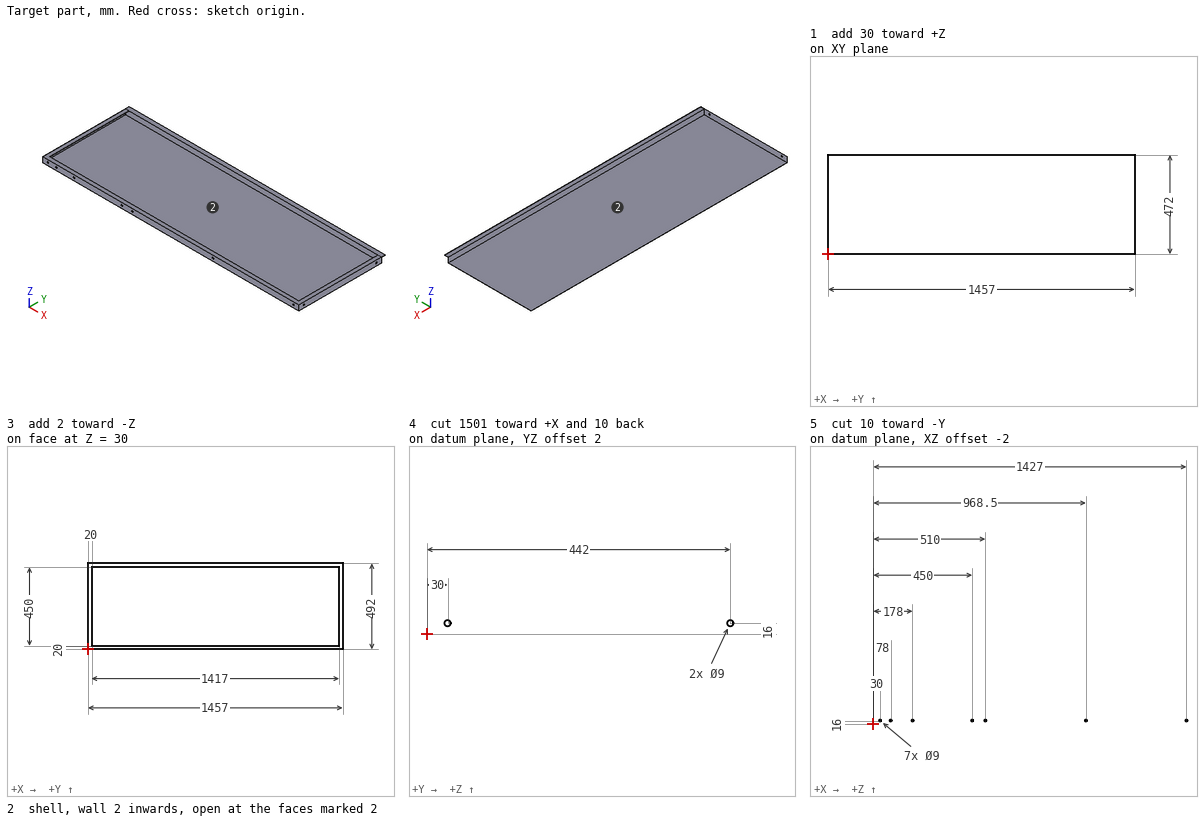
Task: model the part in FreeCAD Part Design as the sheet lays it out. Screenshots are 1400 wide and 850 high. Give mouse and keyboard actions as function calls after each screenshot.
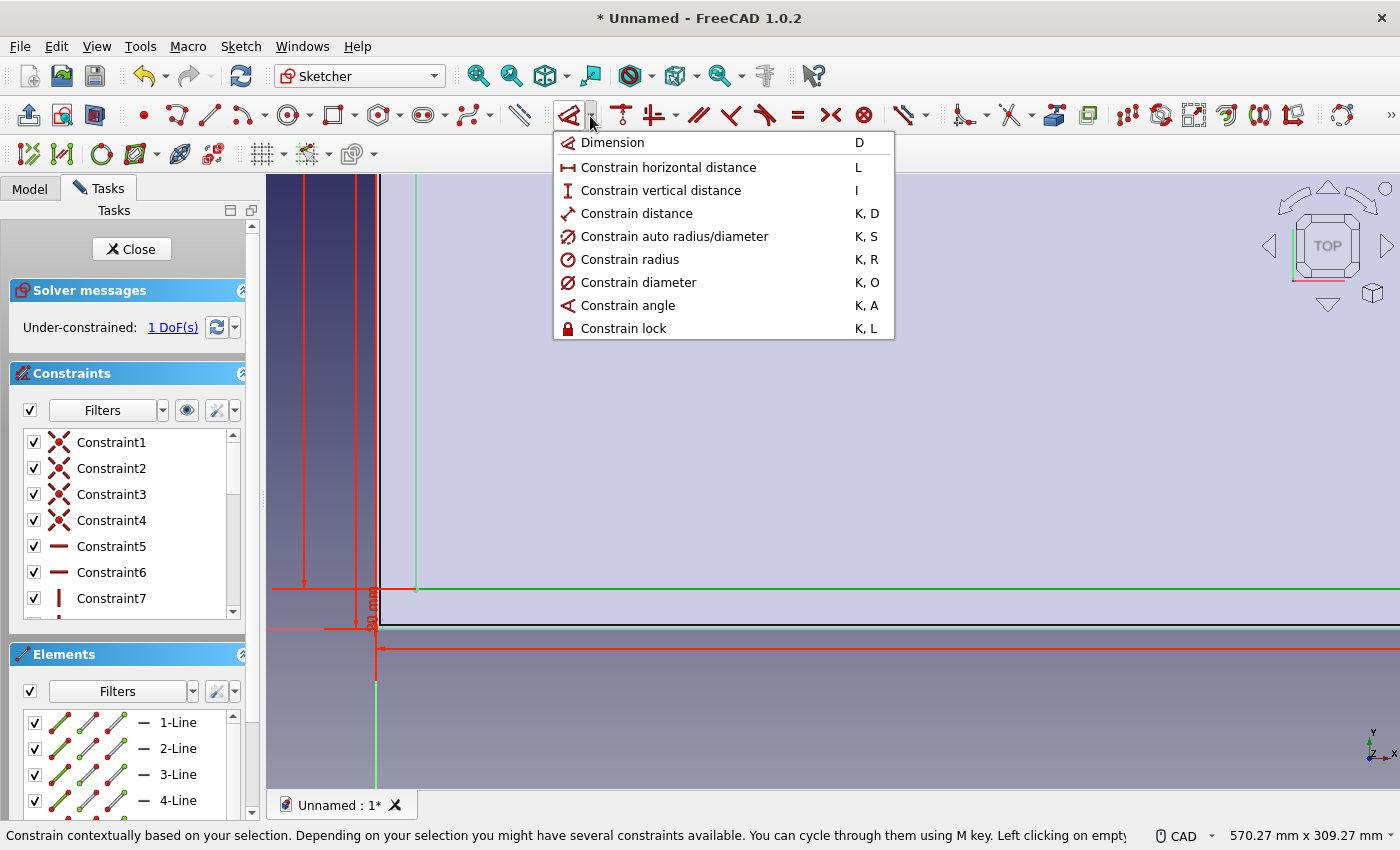
click(724, 168)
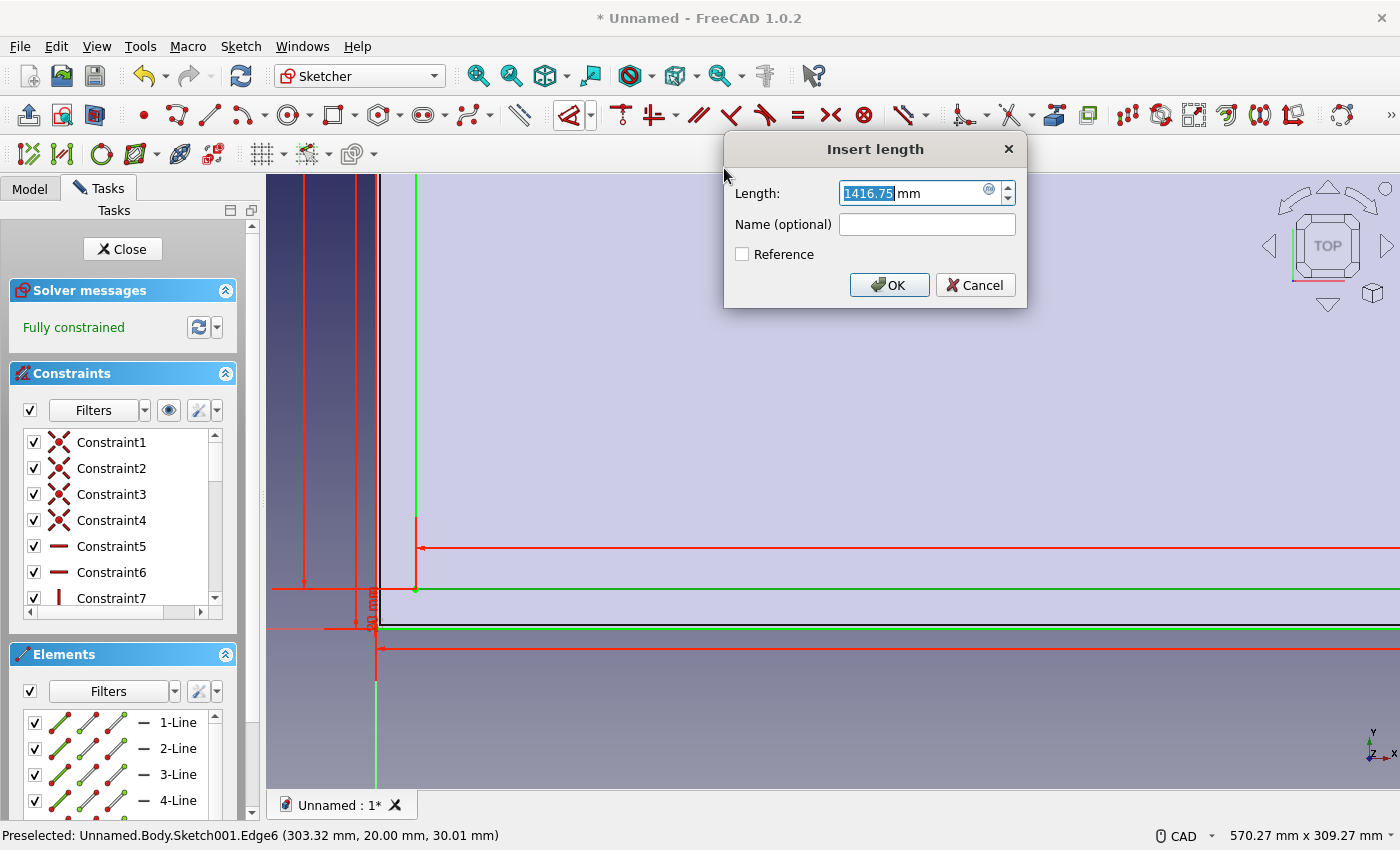
text(1417)
key(Return)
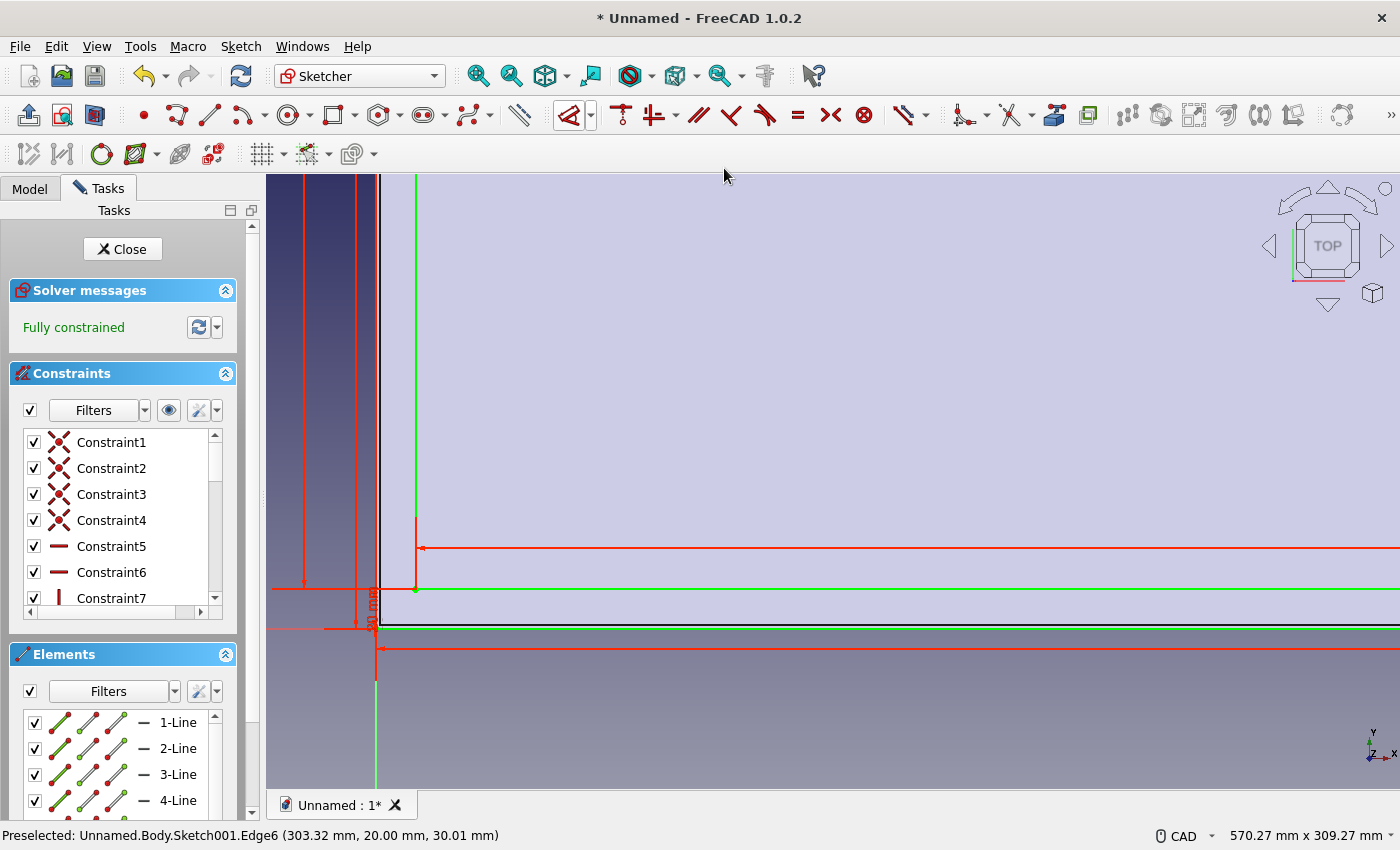
click(123, 249)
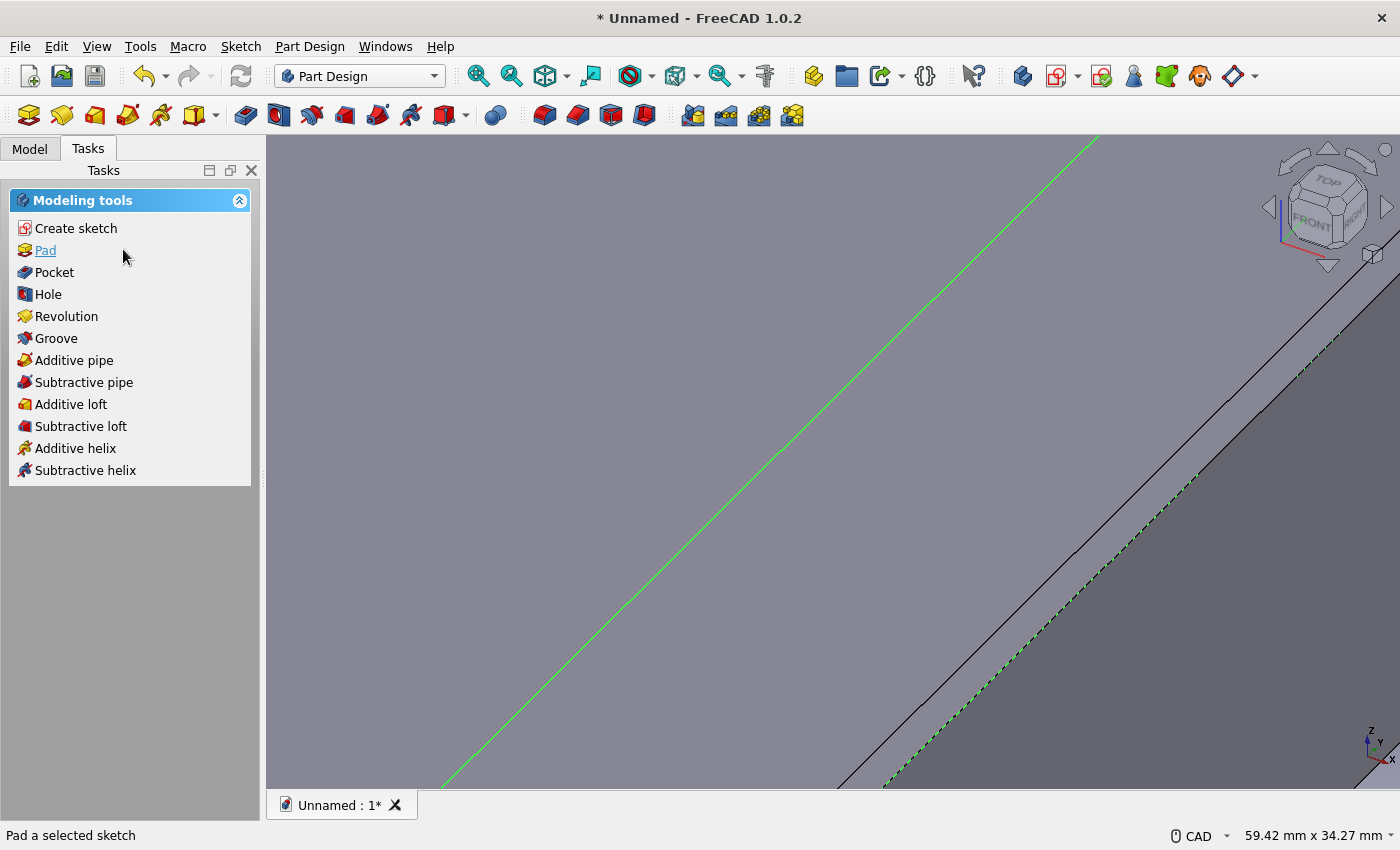
click(29, 116)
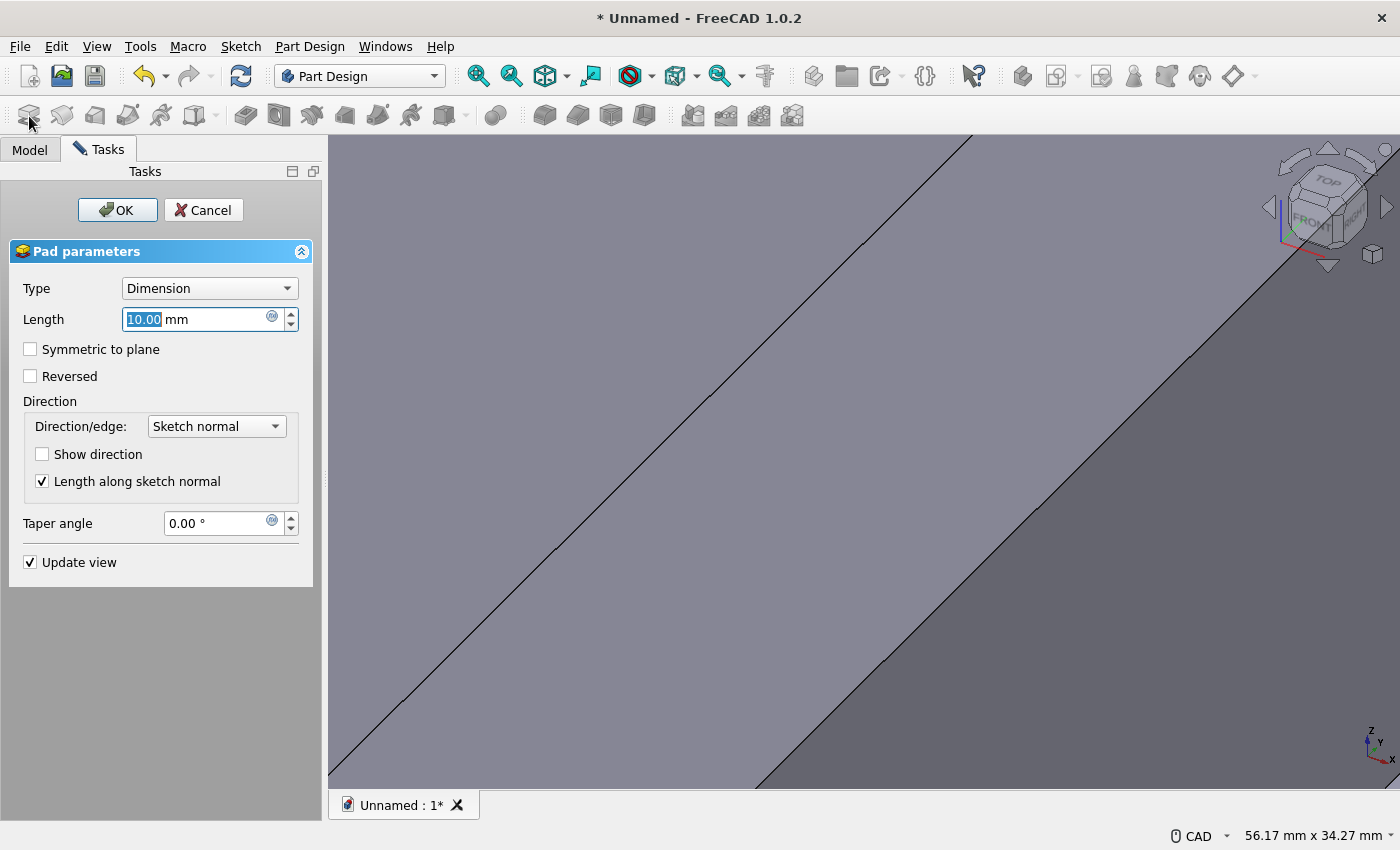
text(2)
key(Tab)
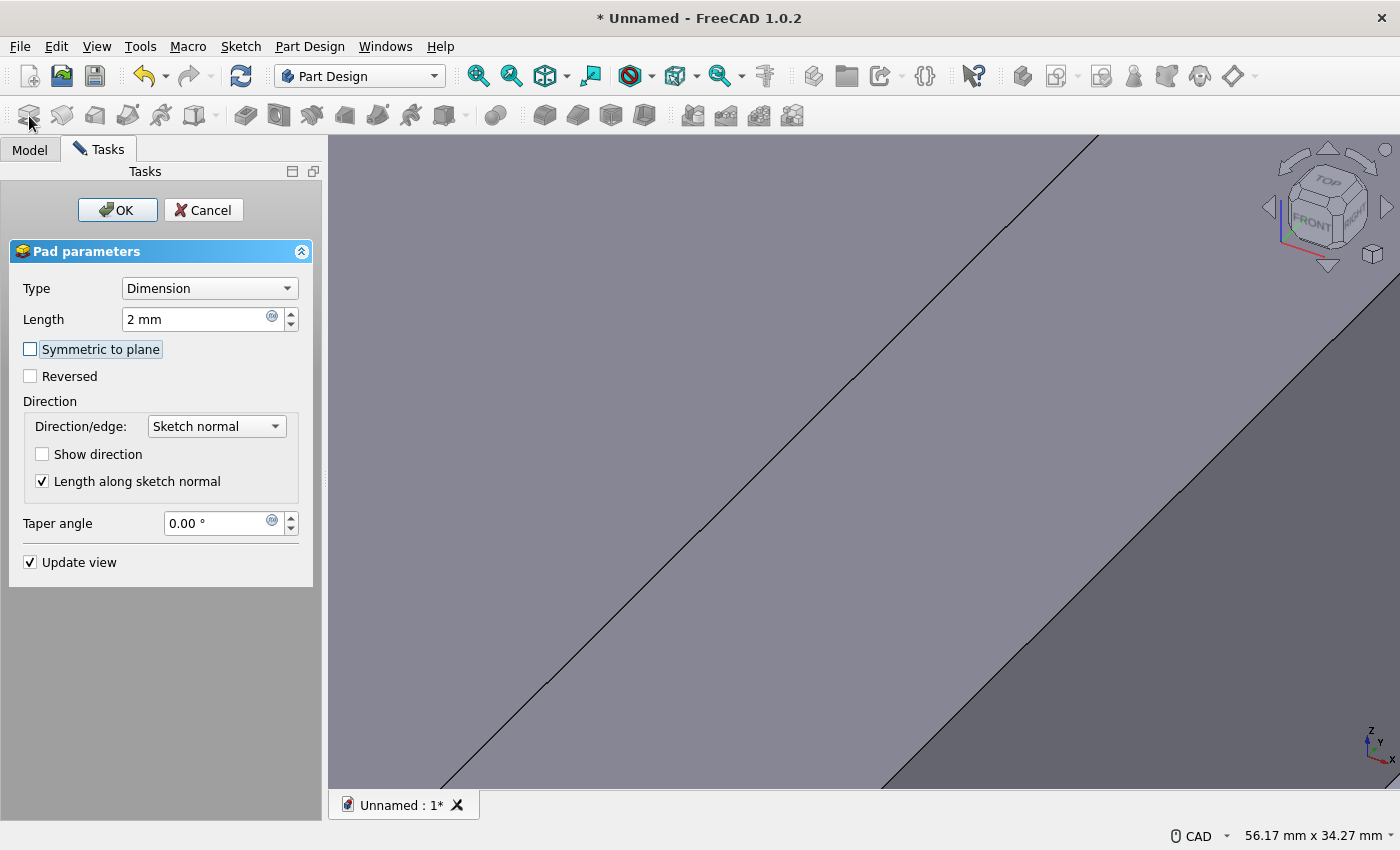
click(31, 376)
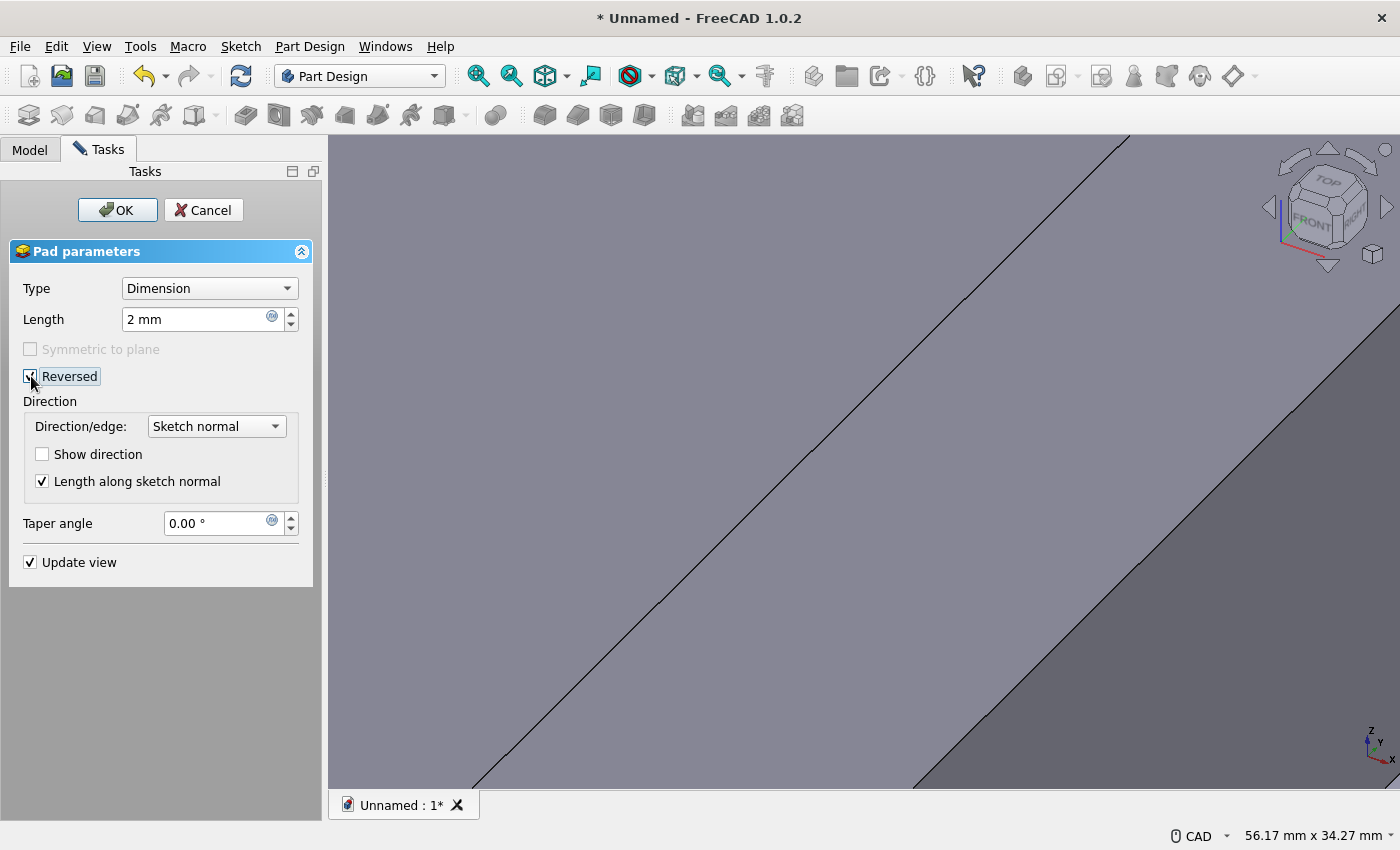
click(118, 210)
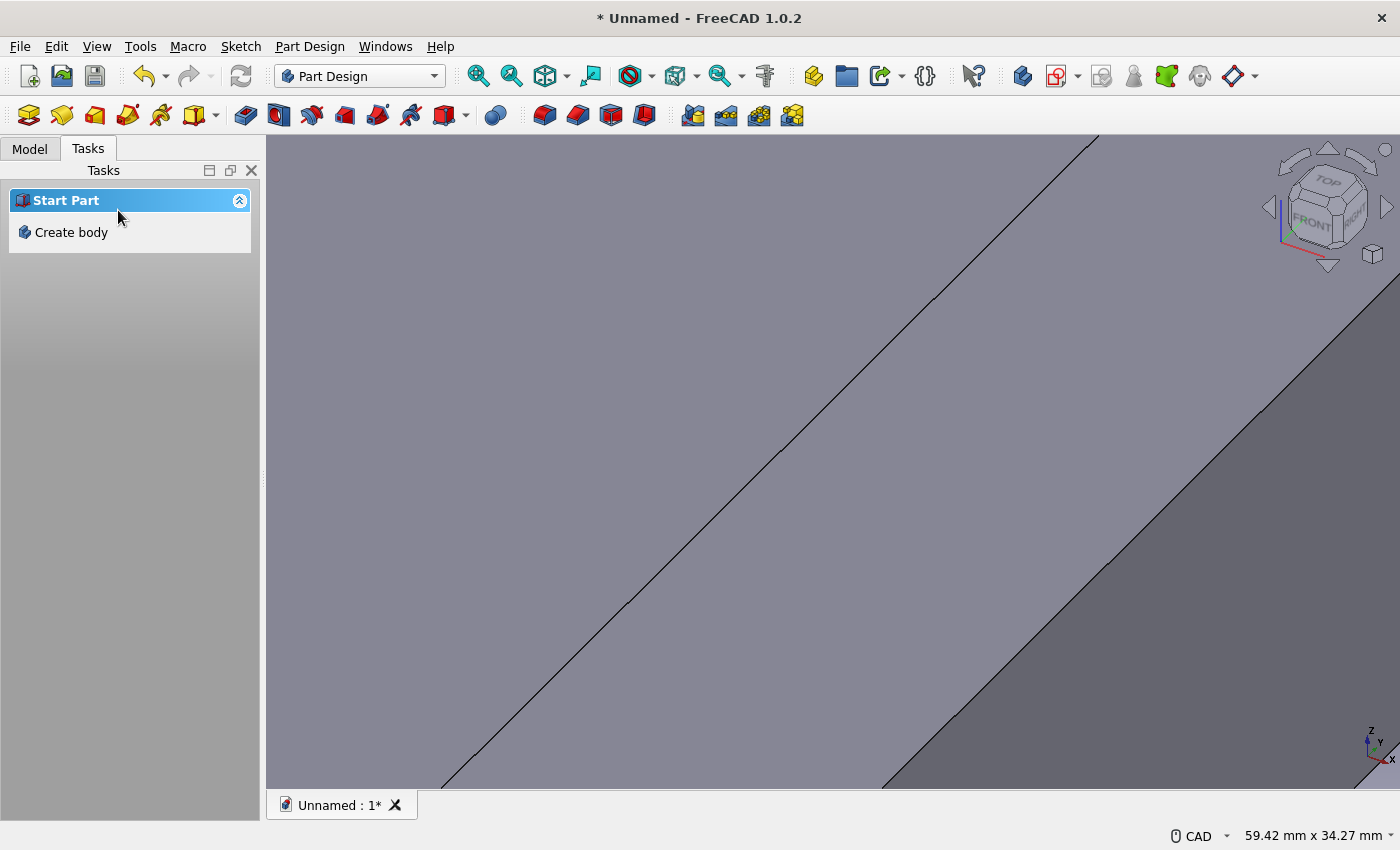
key(v)
key(f)